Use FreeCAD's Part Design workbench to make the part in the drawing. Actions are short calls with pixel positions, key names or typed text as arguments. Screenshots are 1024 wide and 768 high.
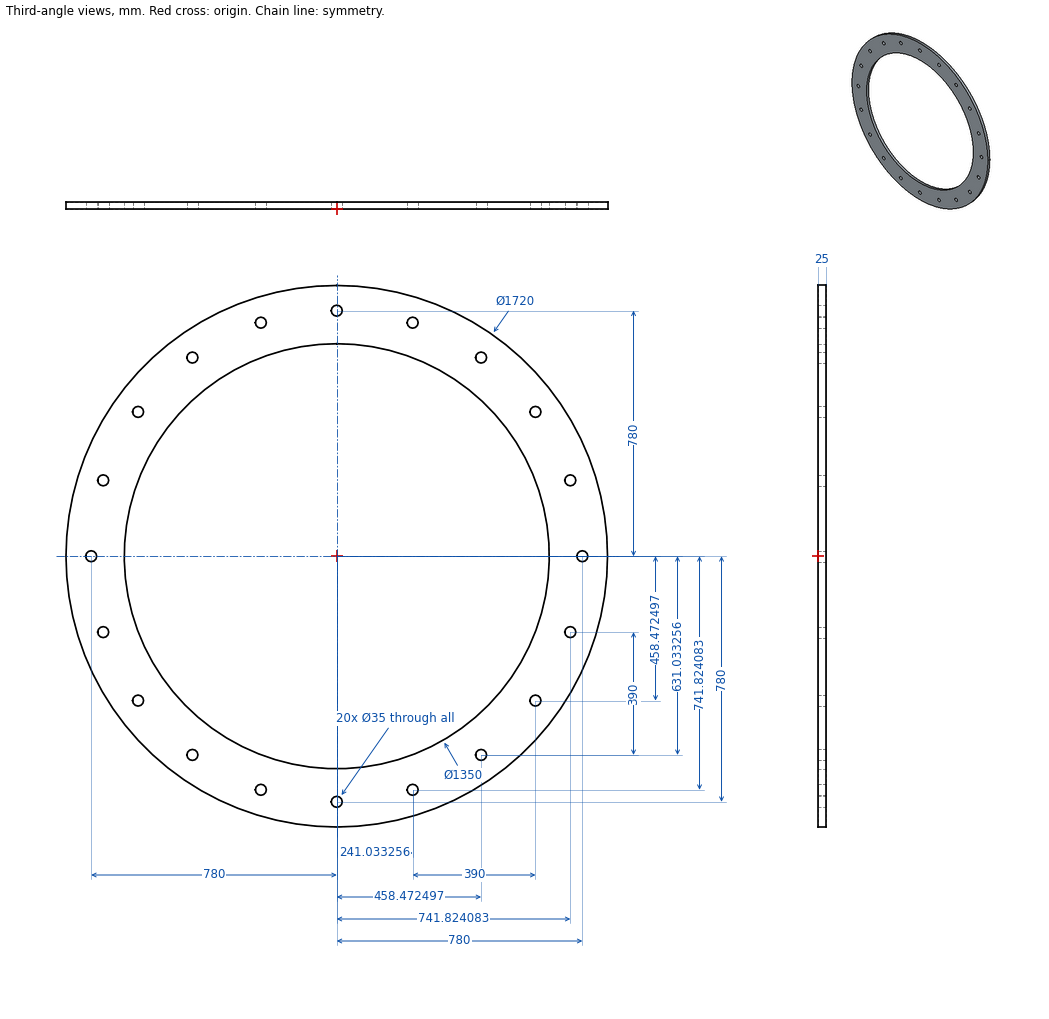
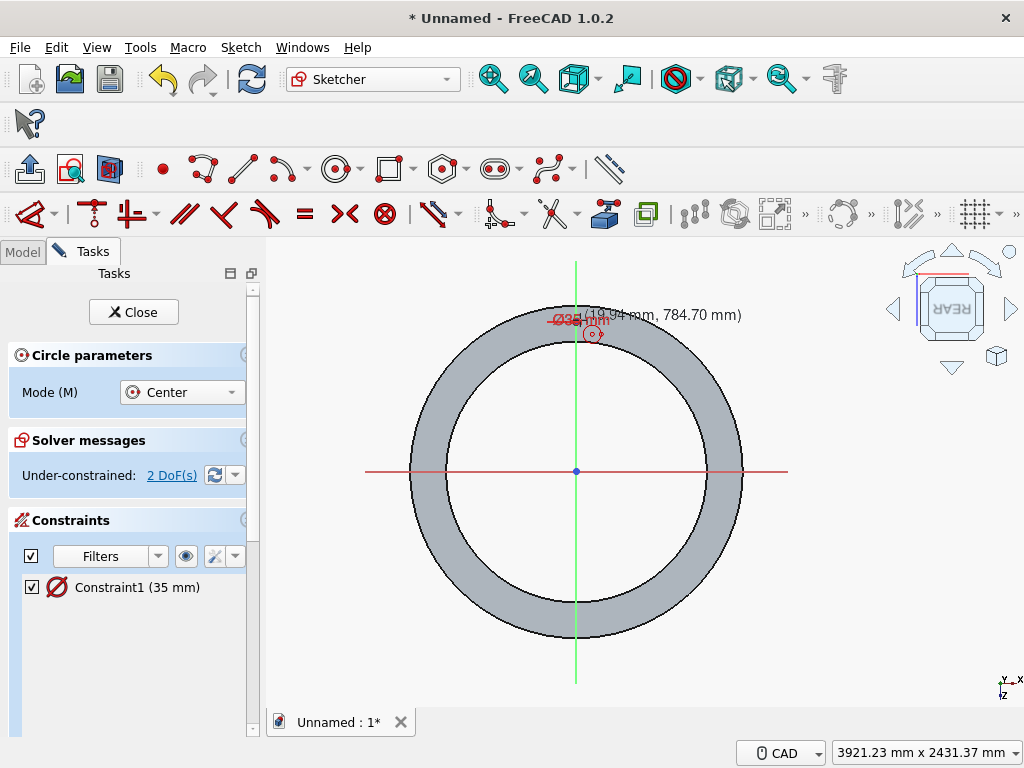
click(623, 329)
move(625, 326)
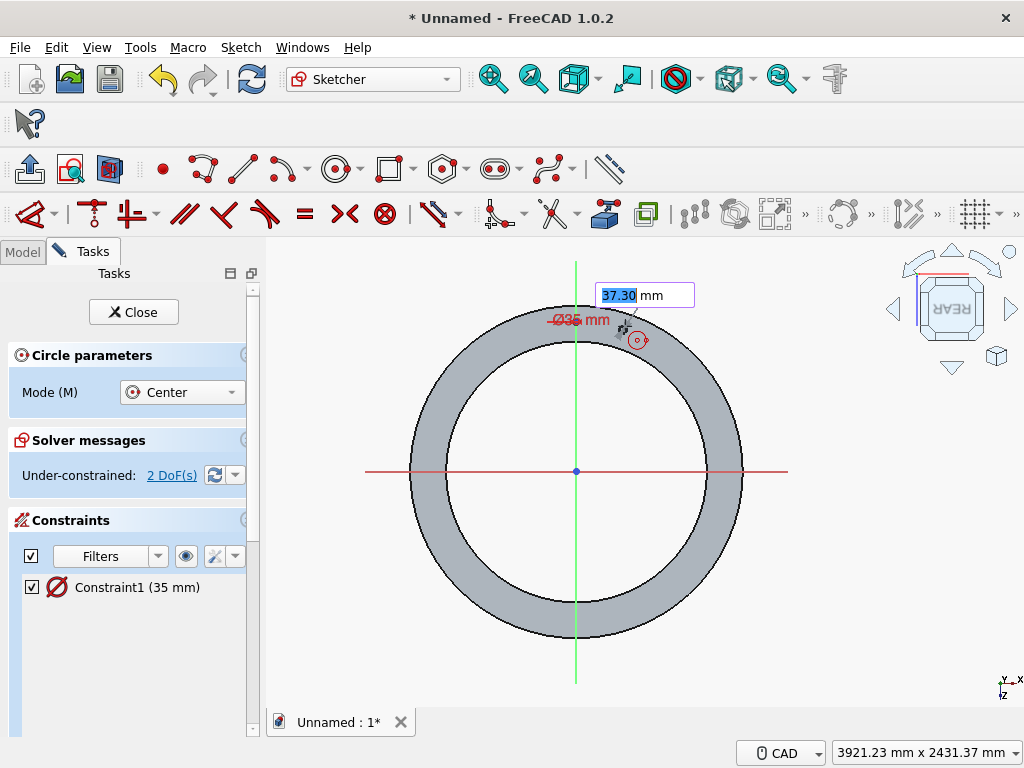
text(35)
key(Return)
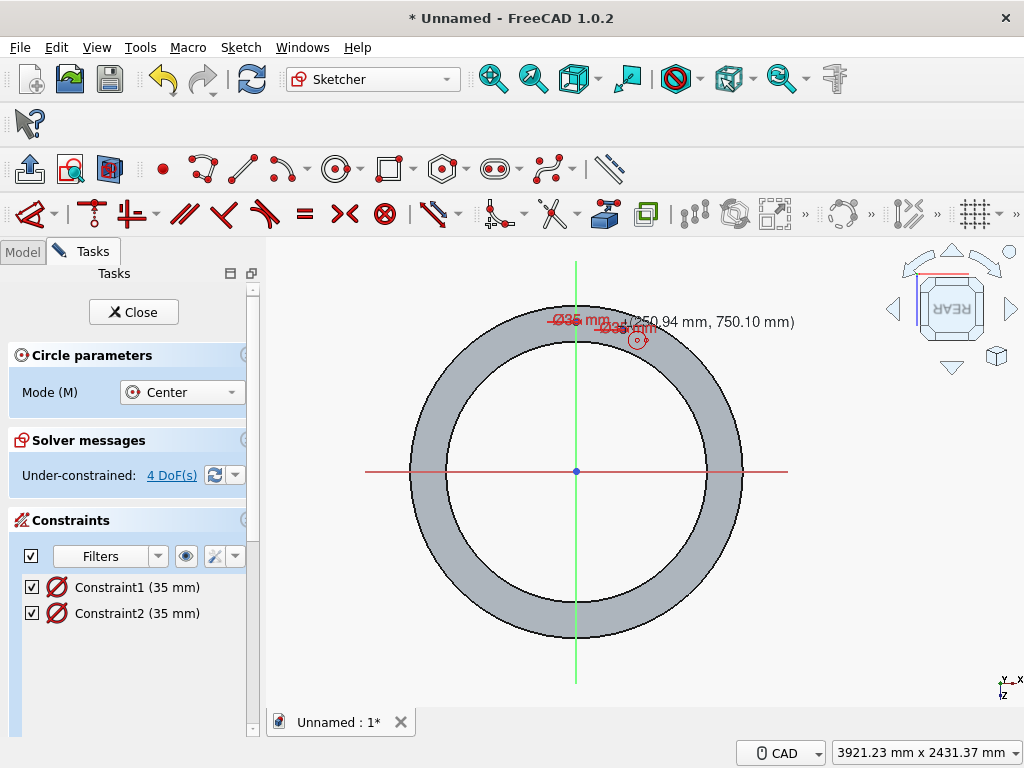
scroll(665, 350, up, 10)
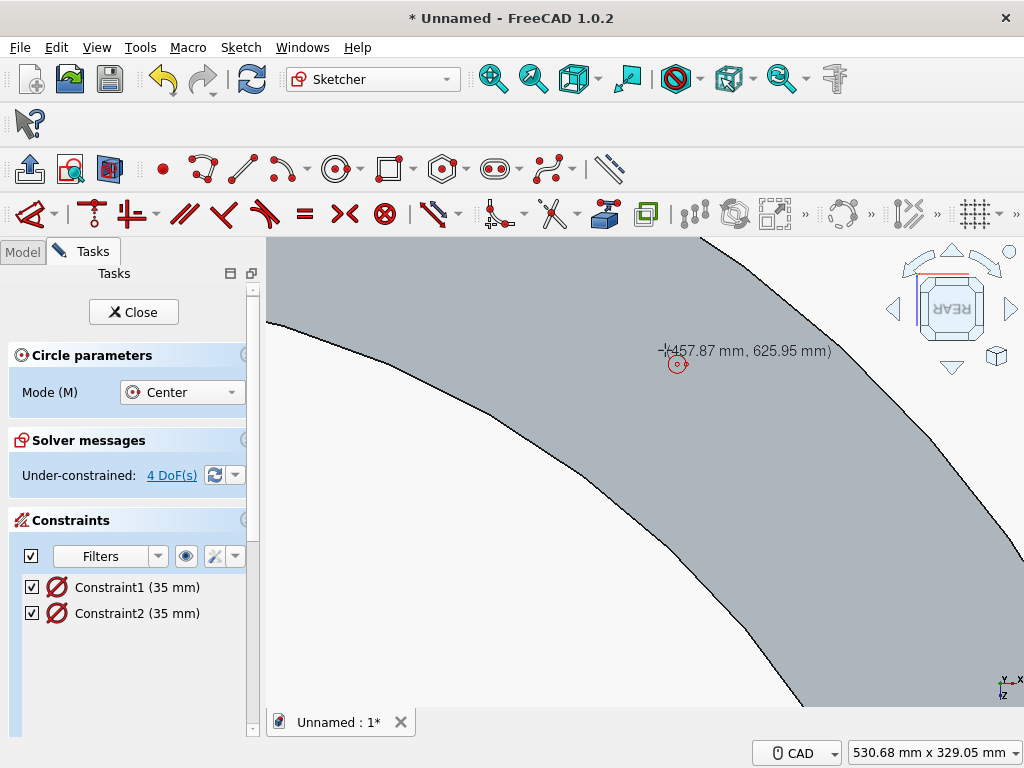
scroll(666, 350, down, 10)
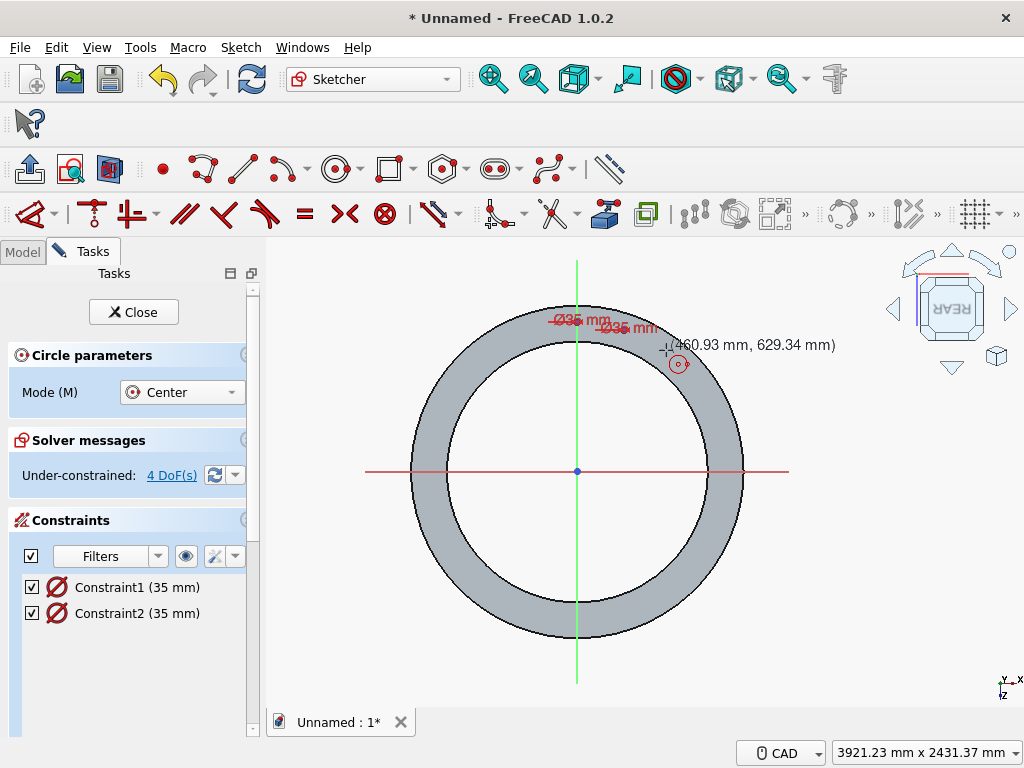
click(666, 350)
move(668, 348)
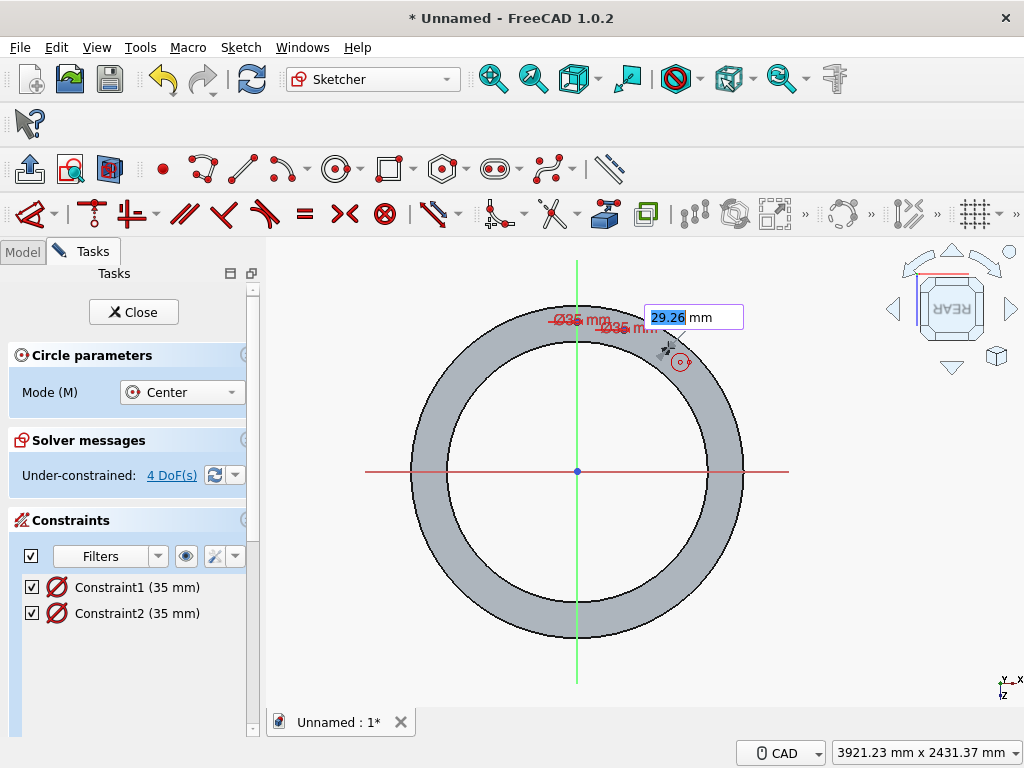
text(35)
key(Return)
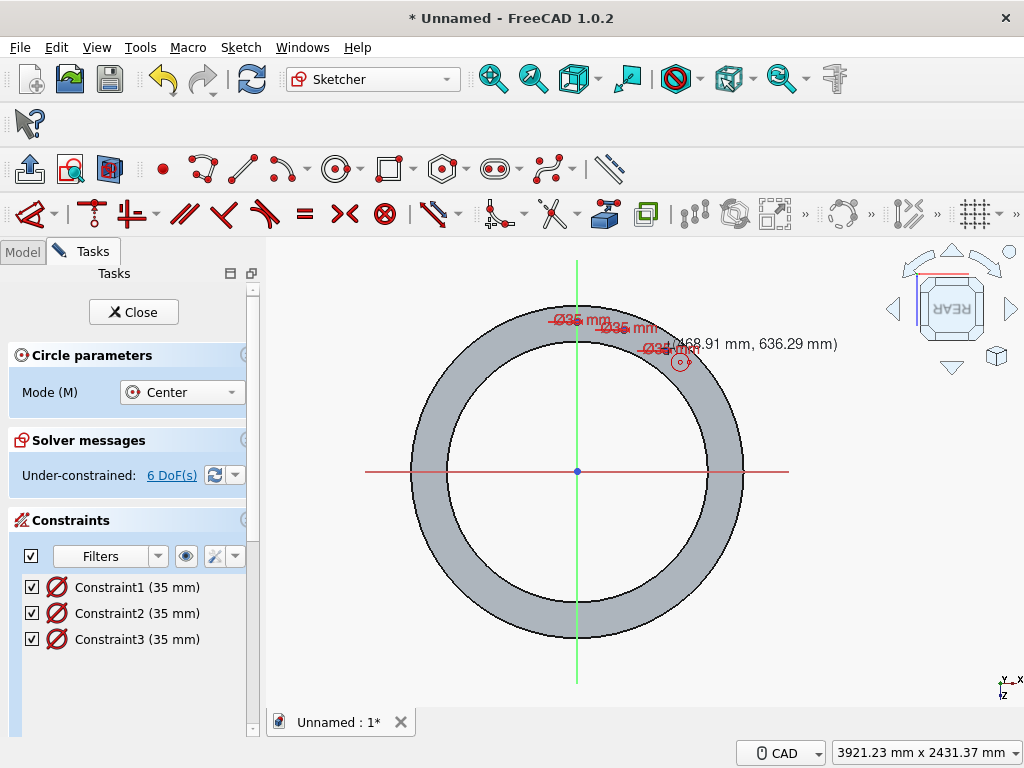
scroll(699, 383, up, 10)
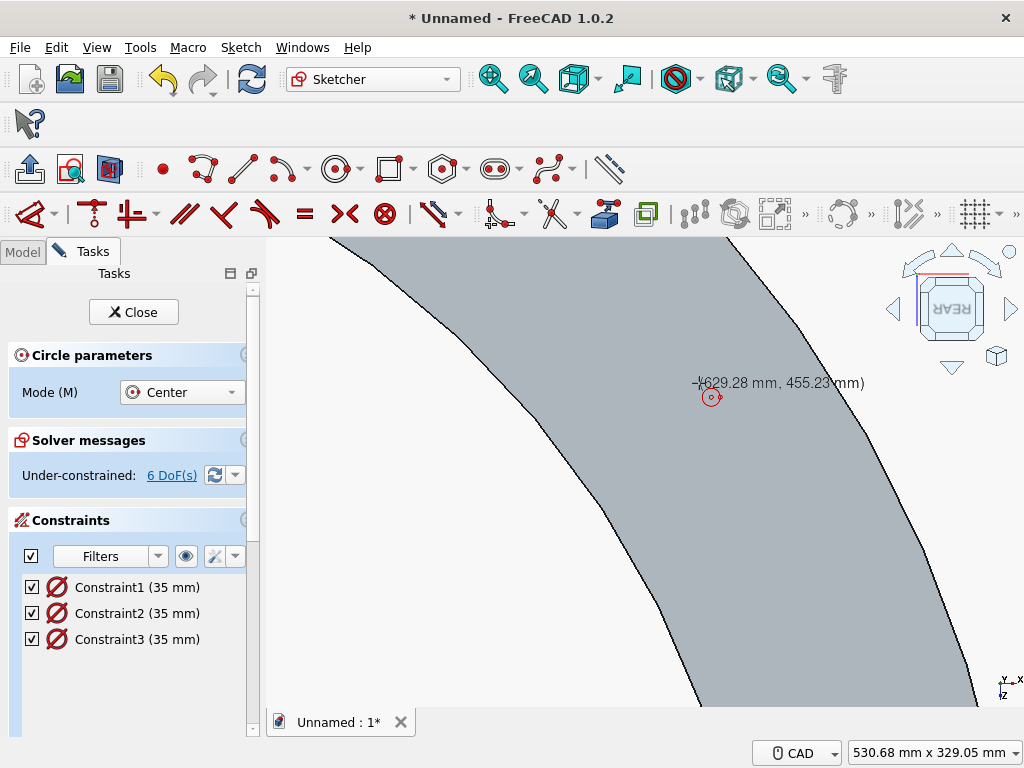
scroll(699, 383, down, 10)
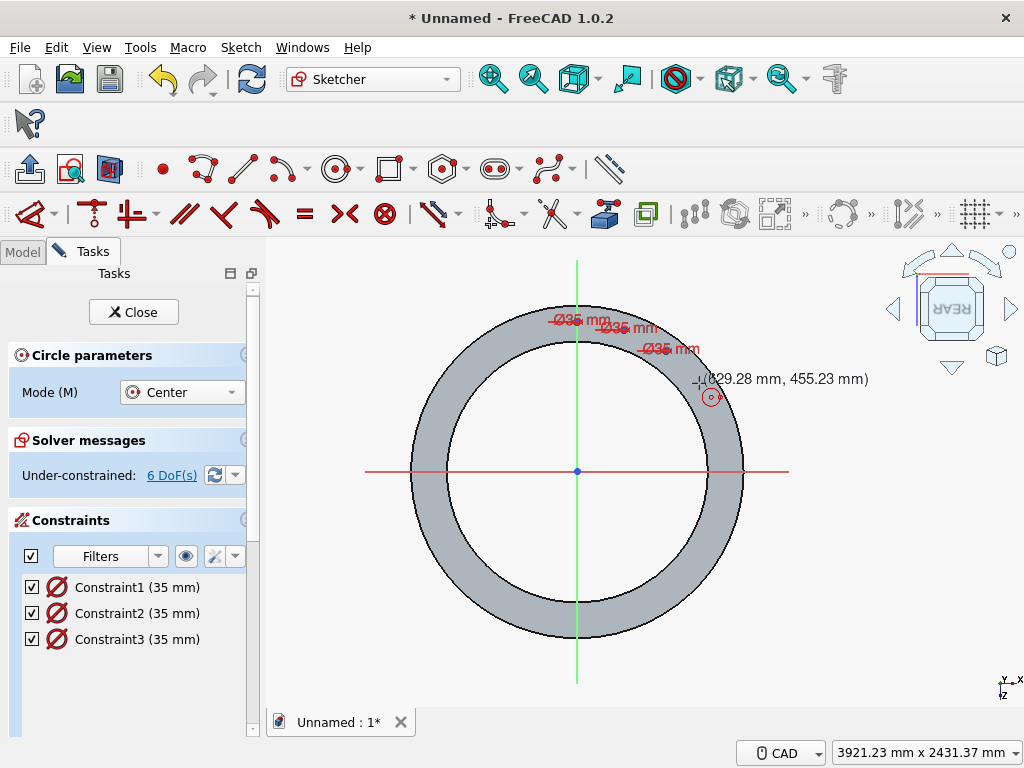
click(699, 383)
move(702, 381)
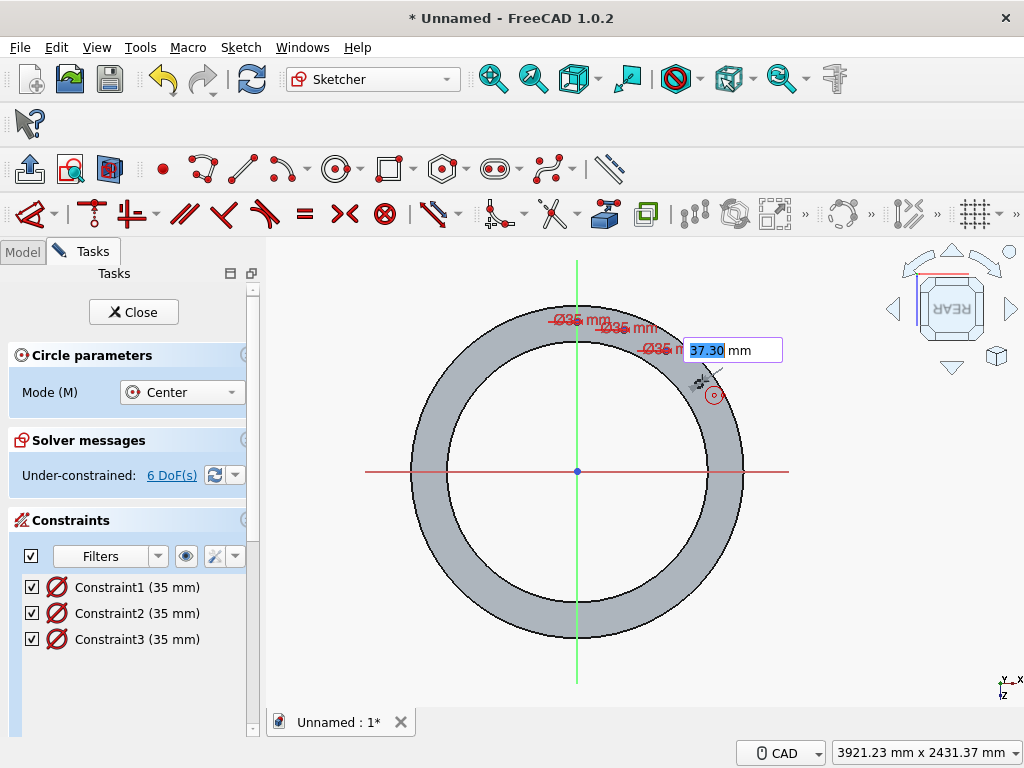
text(35)
key(Return)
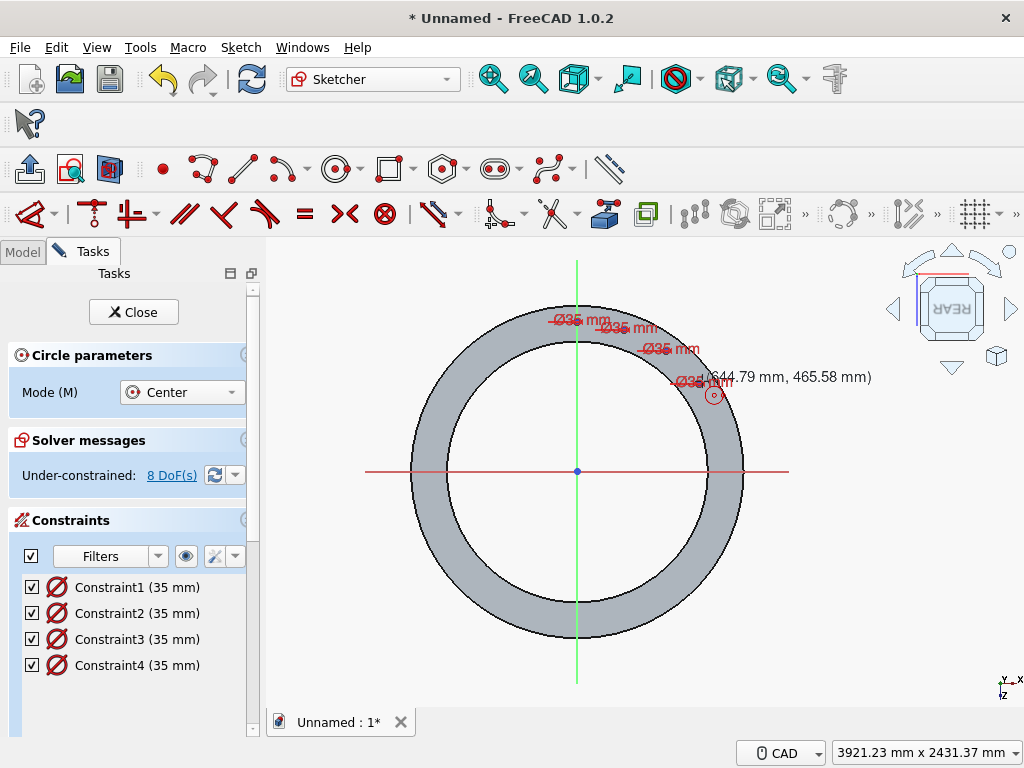
scroll(721, 425, up, 10)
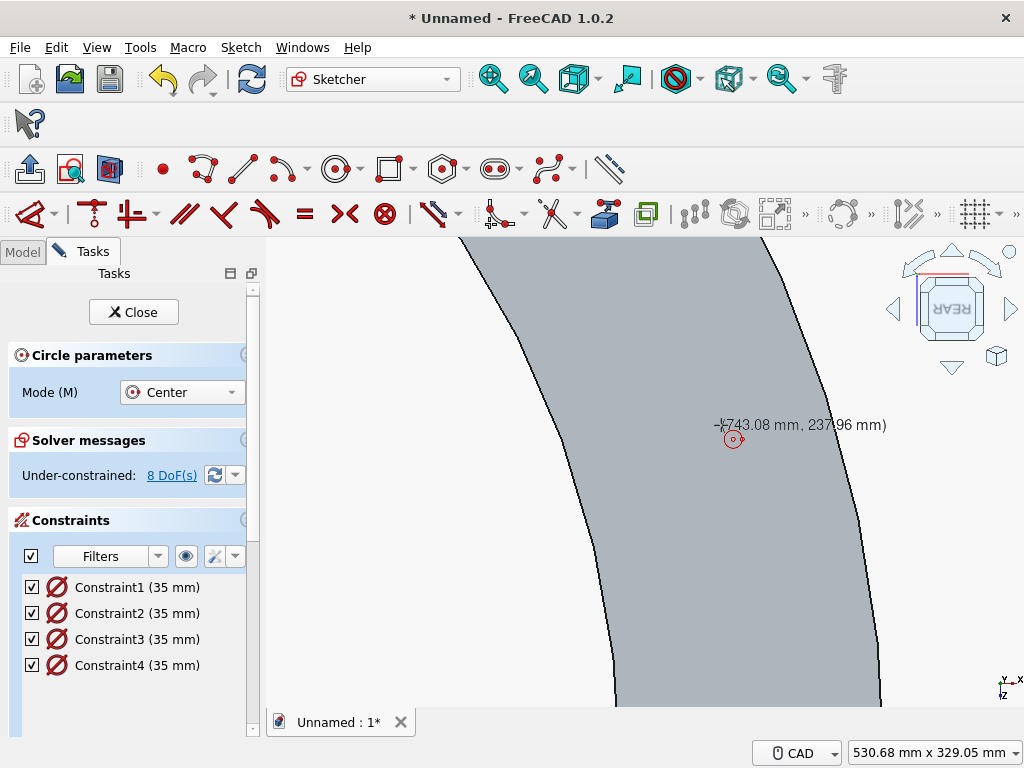
scroll(721, 425, down, 10)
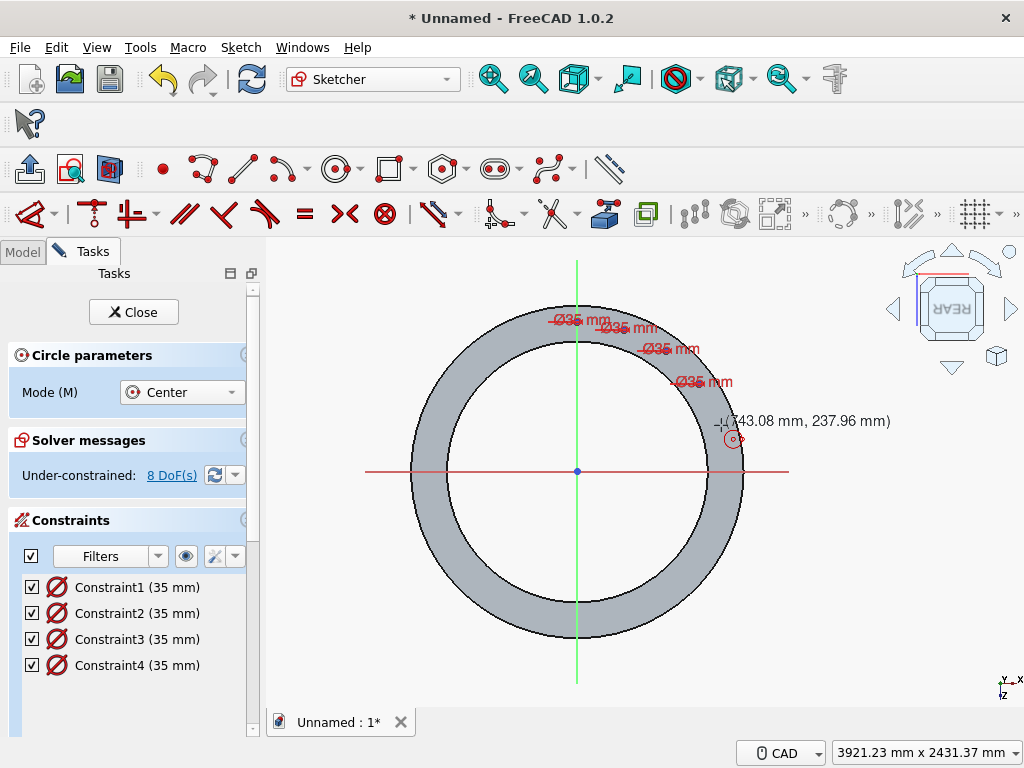
click(721, 425)
move(723, 423)